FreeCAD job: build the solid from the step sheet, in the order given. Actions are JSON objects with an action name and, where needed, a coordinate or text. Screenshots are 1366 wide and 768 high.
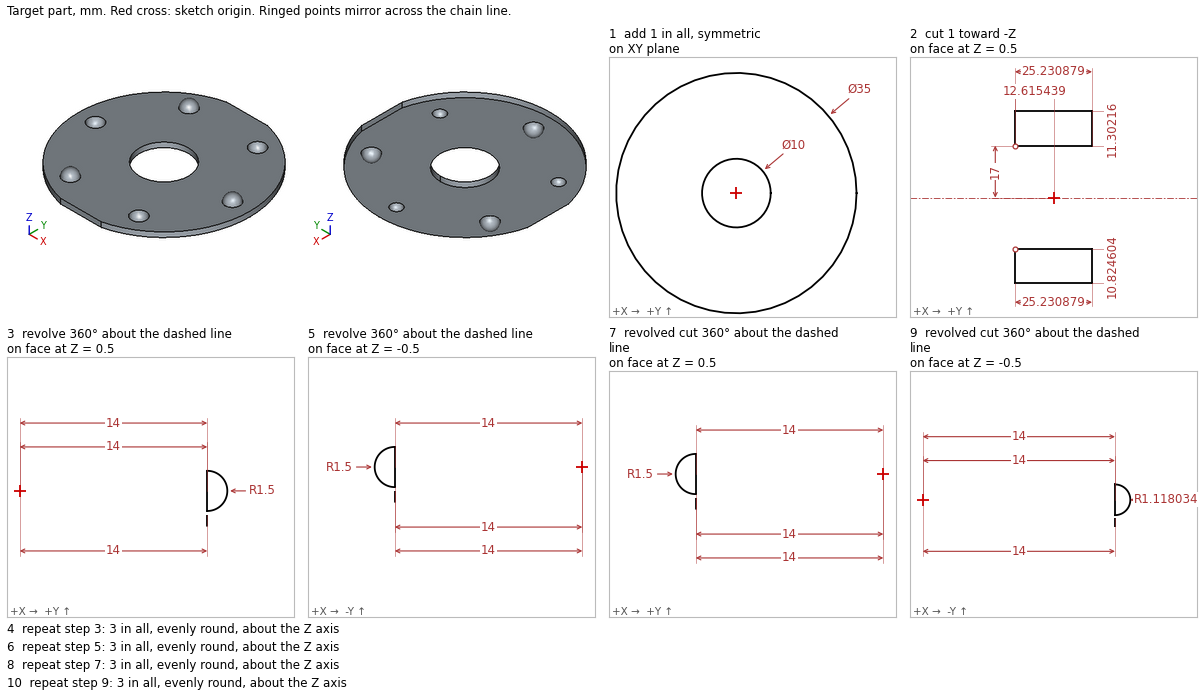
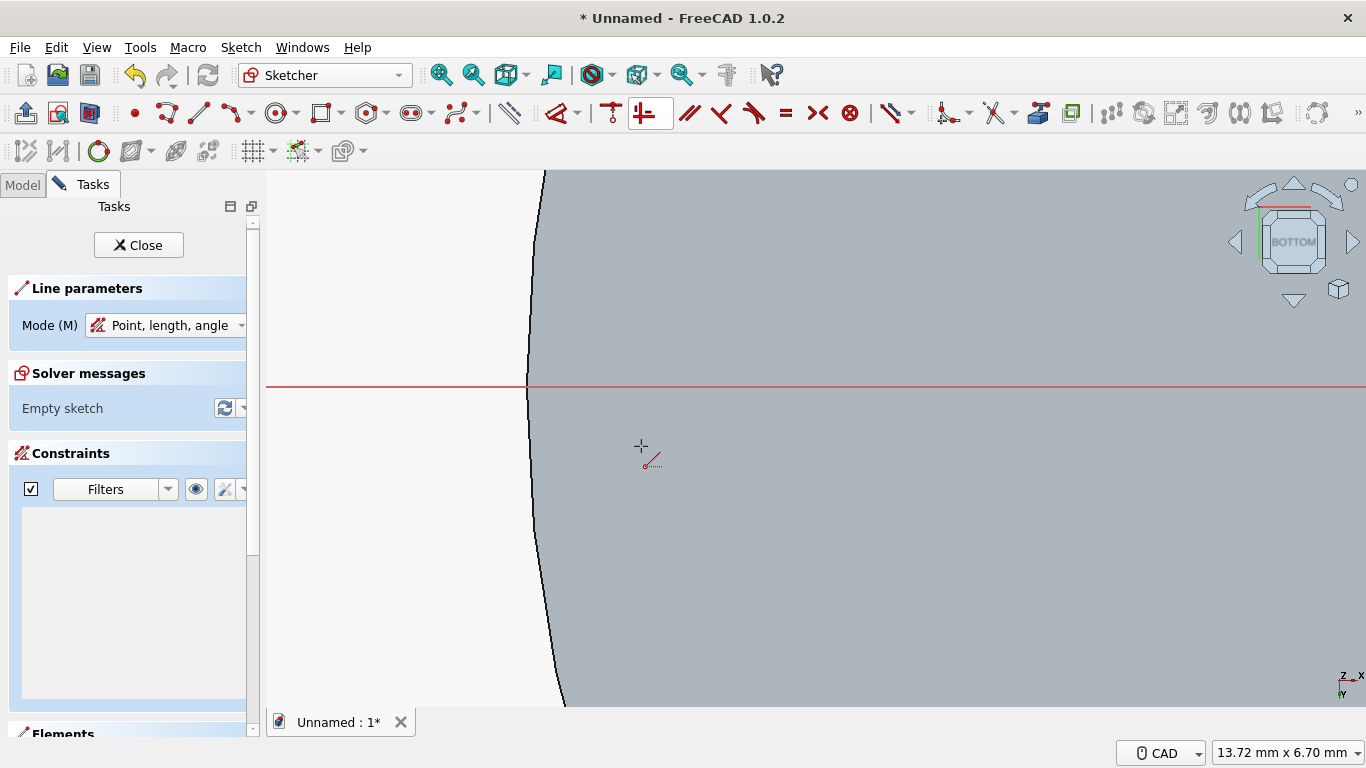
{"action": "left_click", "coordinate": [807, 507]}
{"action": "left_click", "coordinate": [807, 266]}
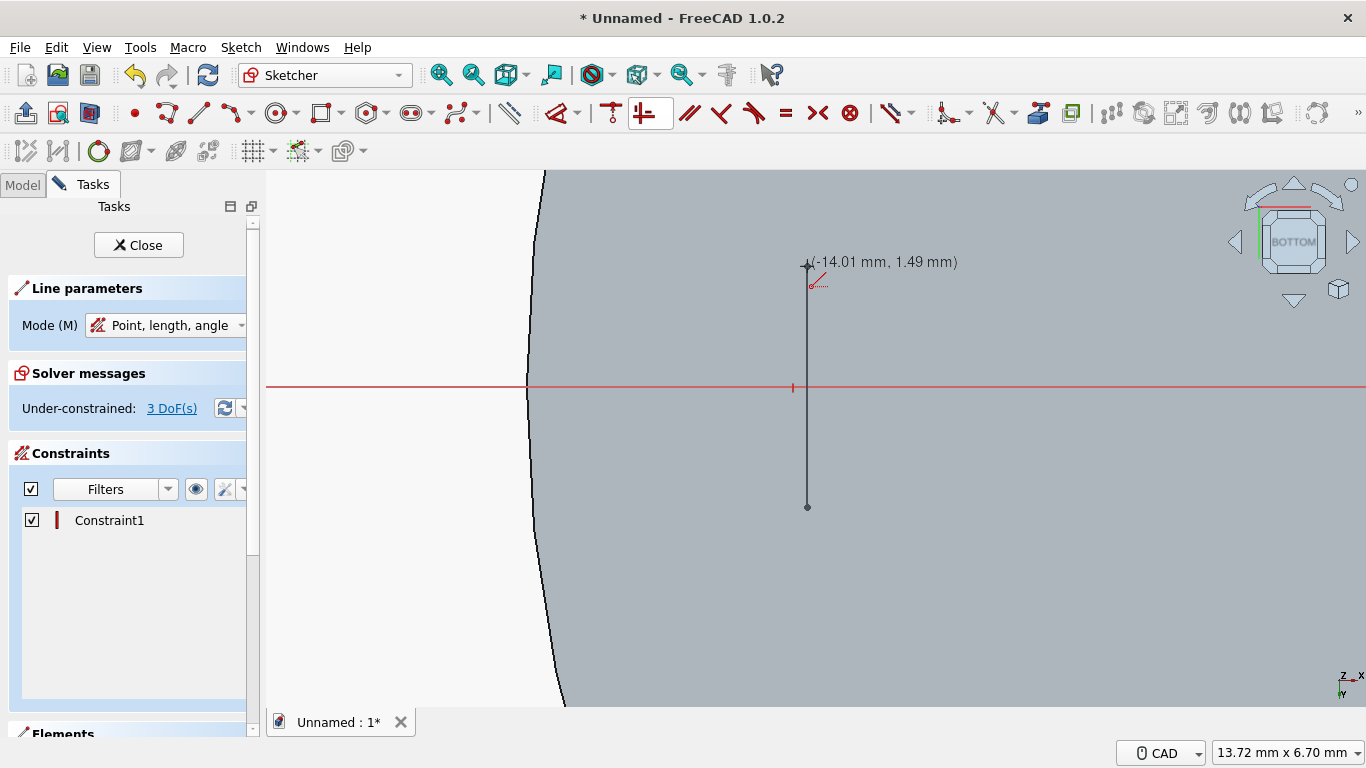
{"action": "left_click", "coordinate": [232, 114]}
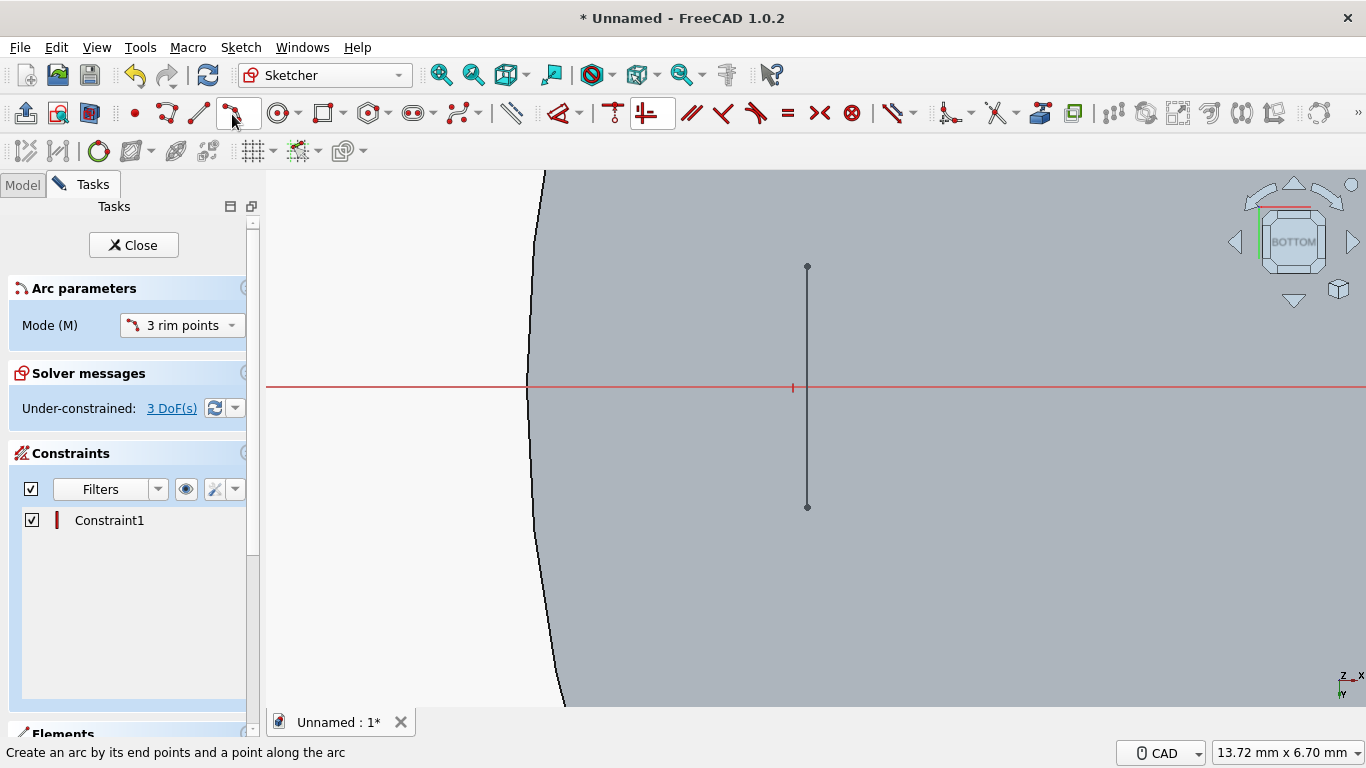
{"action": "left_click", "coordinate": [807, 267]}
{"action": "left_click", "coordinate": [807, 508]}
{"action": "left_click", "coordinate": [693, 349]}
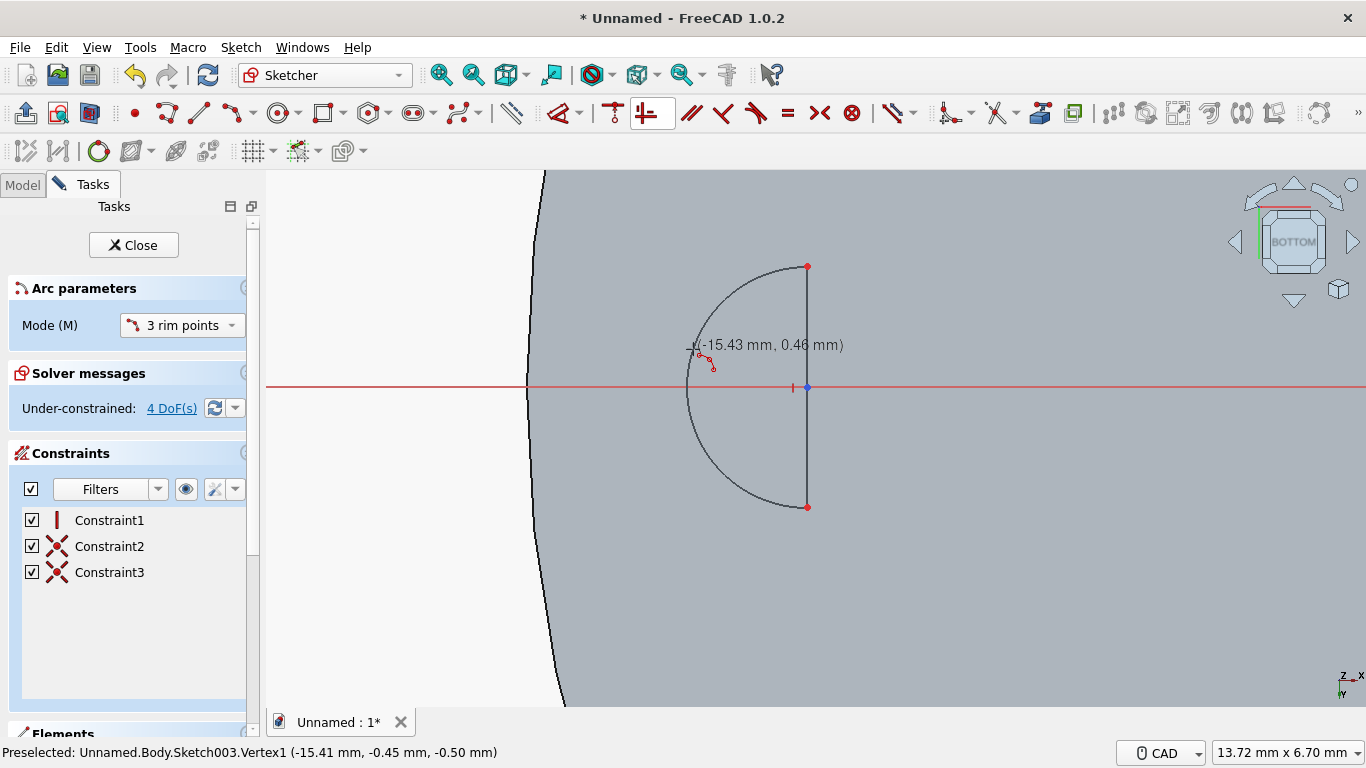
{"action": "left_click", "coordinate": [200, 114]}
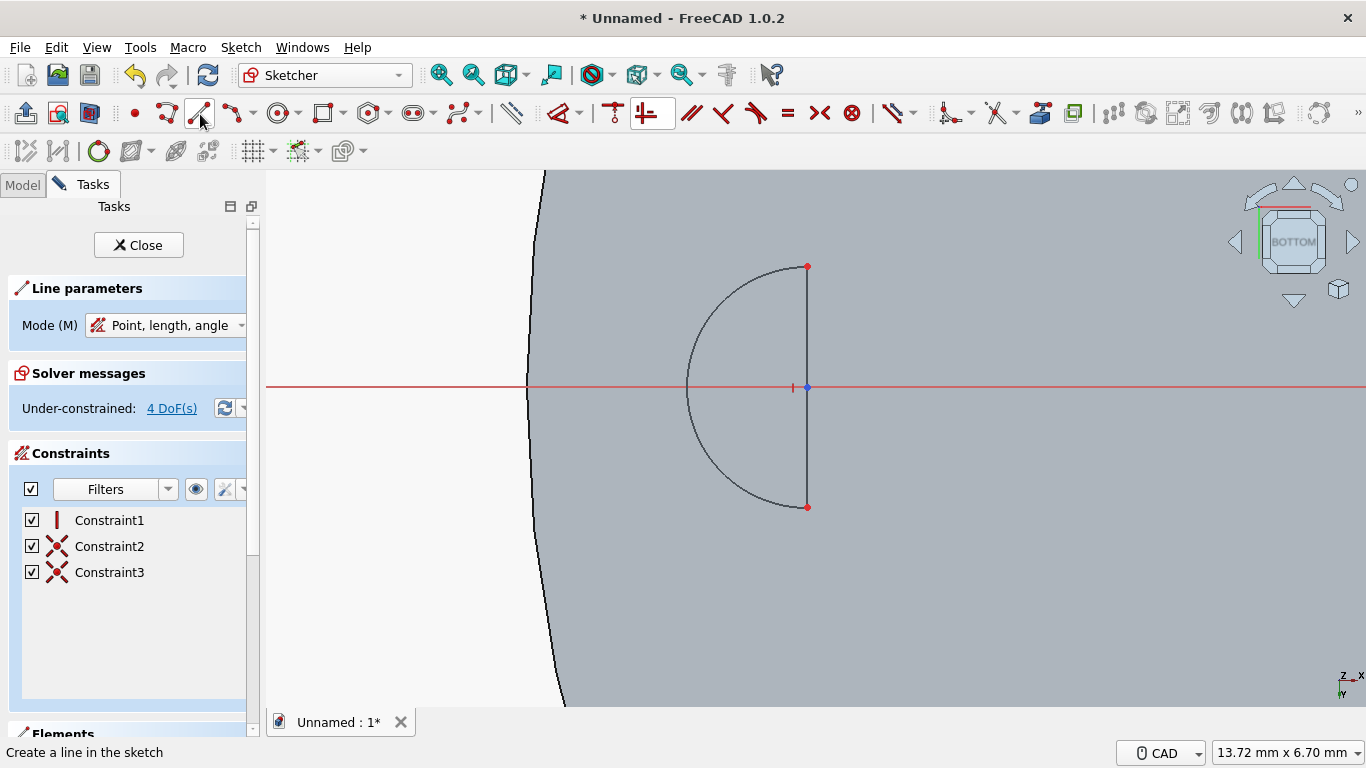
{"action": "left_click", "coordinate": [807, 531]}
{"action": "left_click", "coordinate": [807, 603]}
{"action": "key", "text": "Escape"}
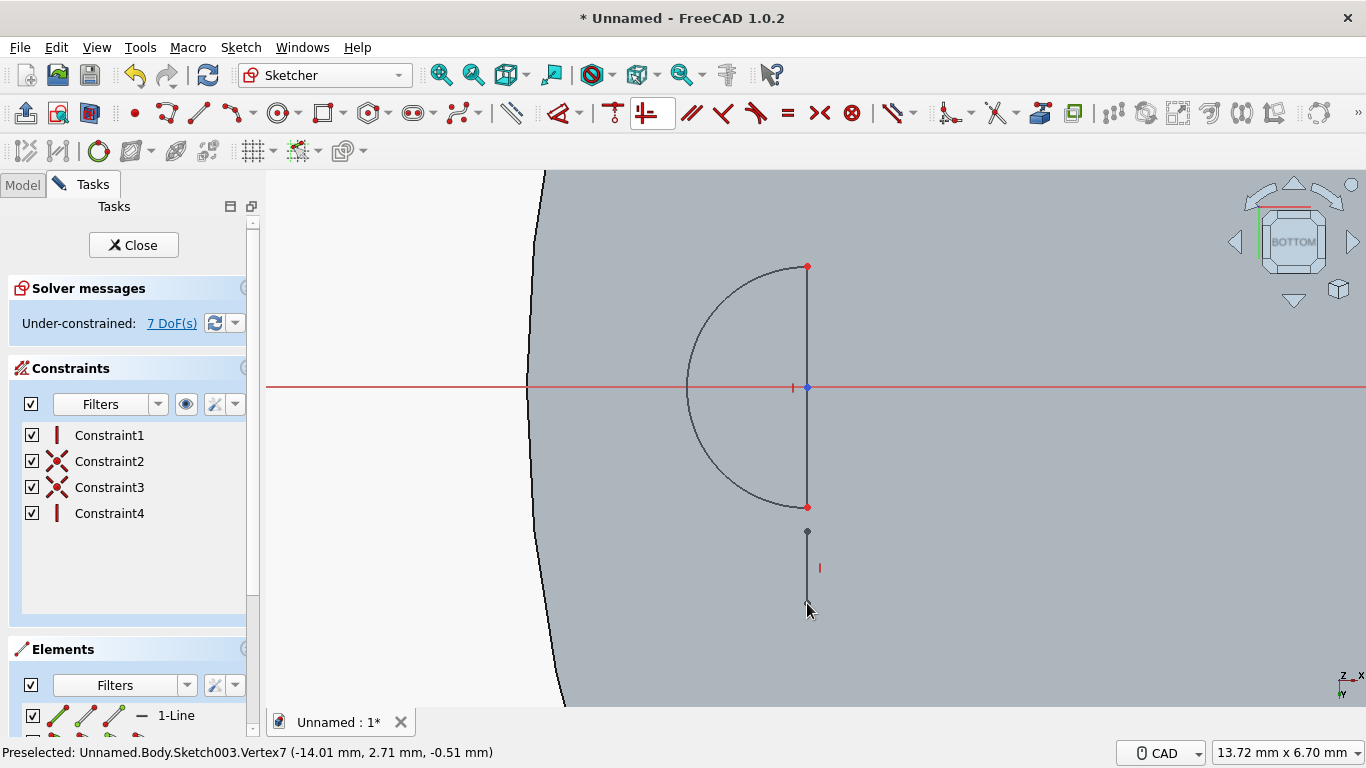
{"action": "left_click", "coordinate": [807, 554]}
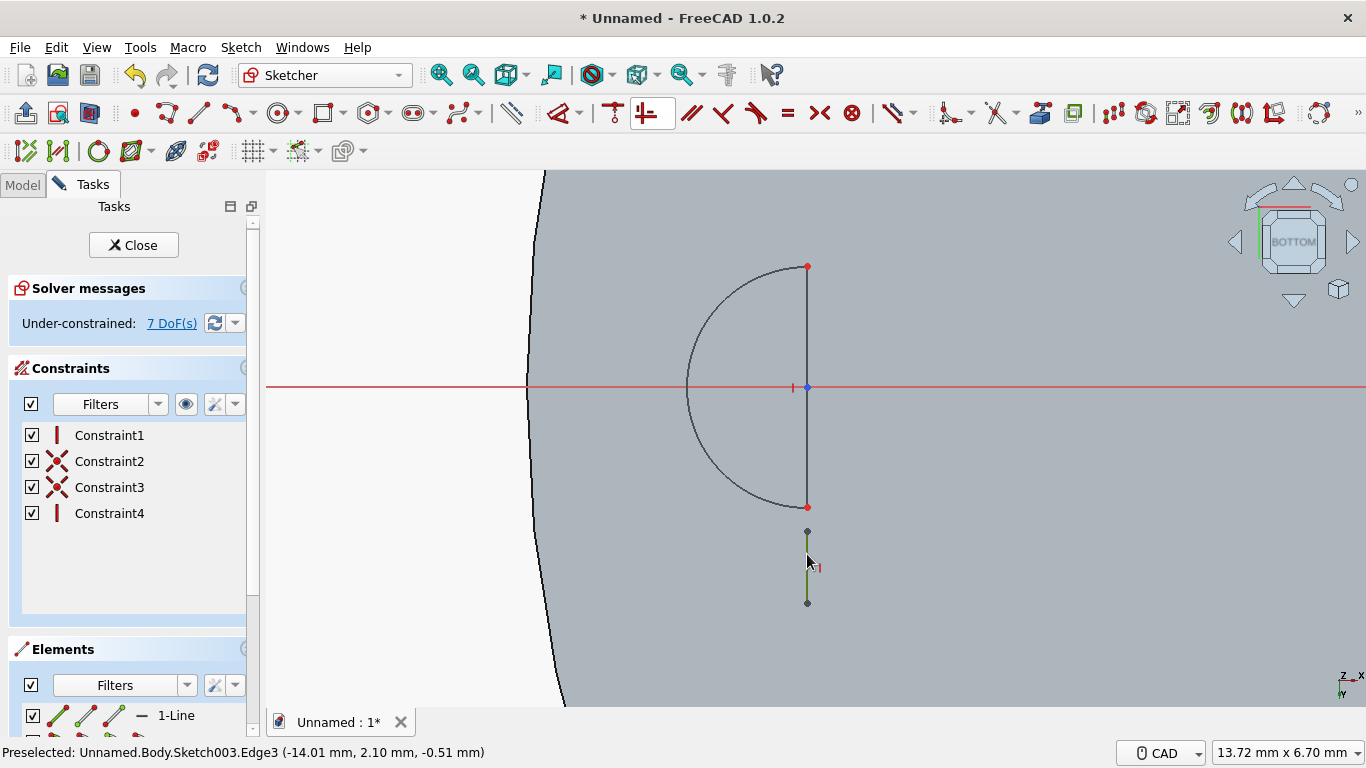
{"action": "key", "text": "g n"}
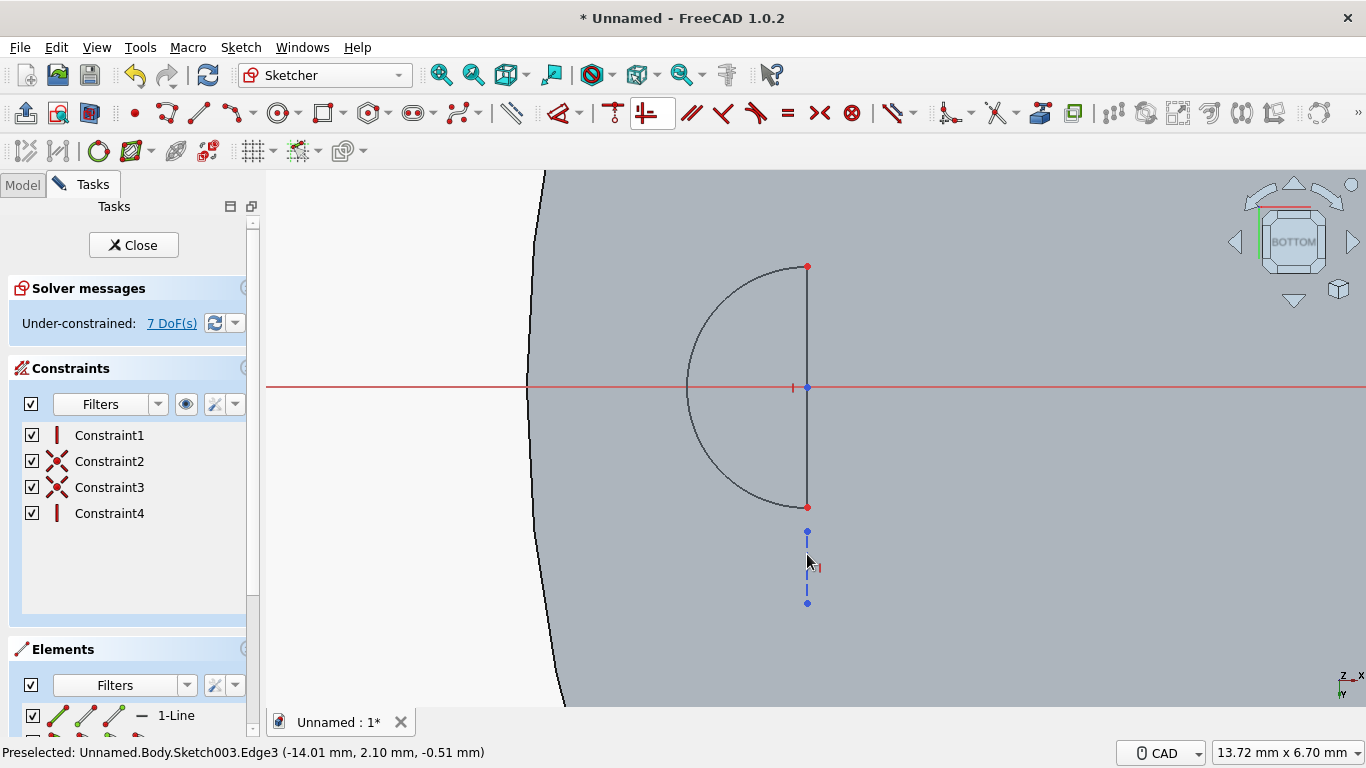
{"action": "left_click", "coordinate": [808, 387]}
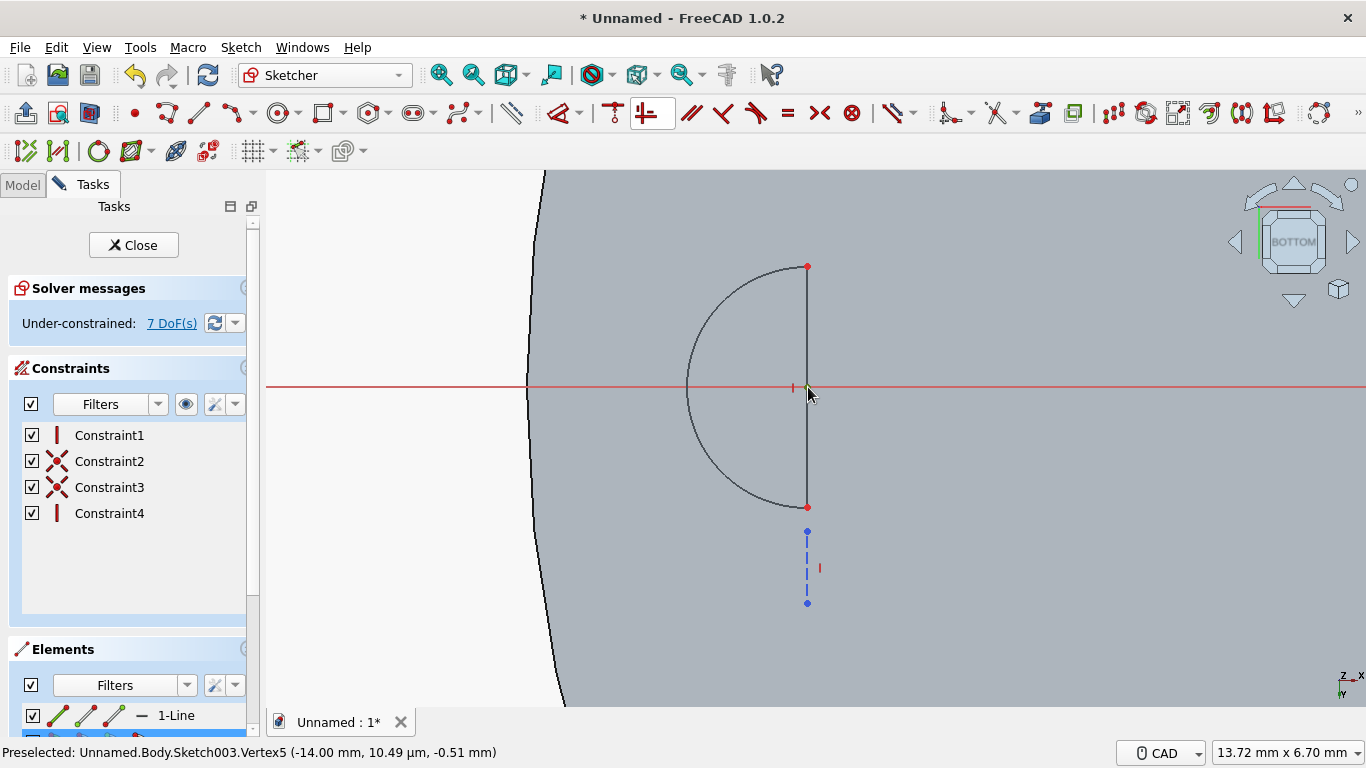
{"action": "left_click", "coordinate": [359, 387]}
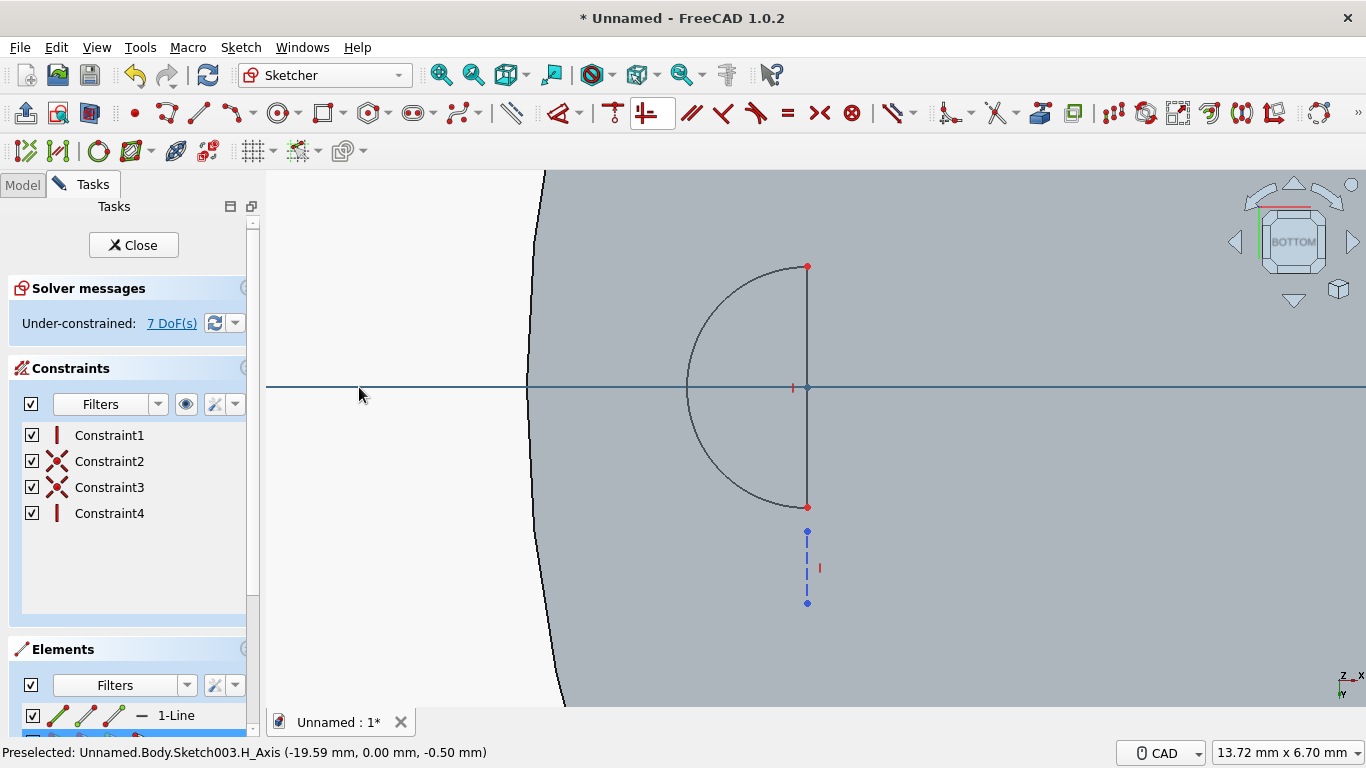
{"action": "key", "text": "c"}